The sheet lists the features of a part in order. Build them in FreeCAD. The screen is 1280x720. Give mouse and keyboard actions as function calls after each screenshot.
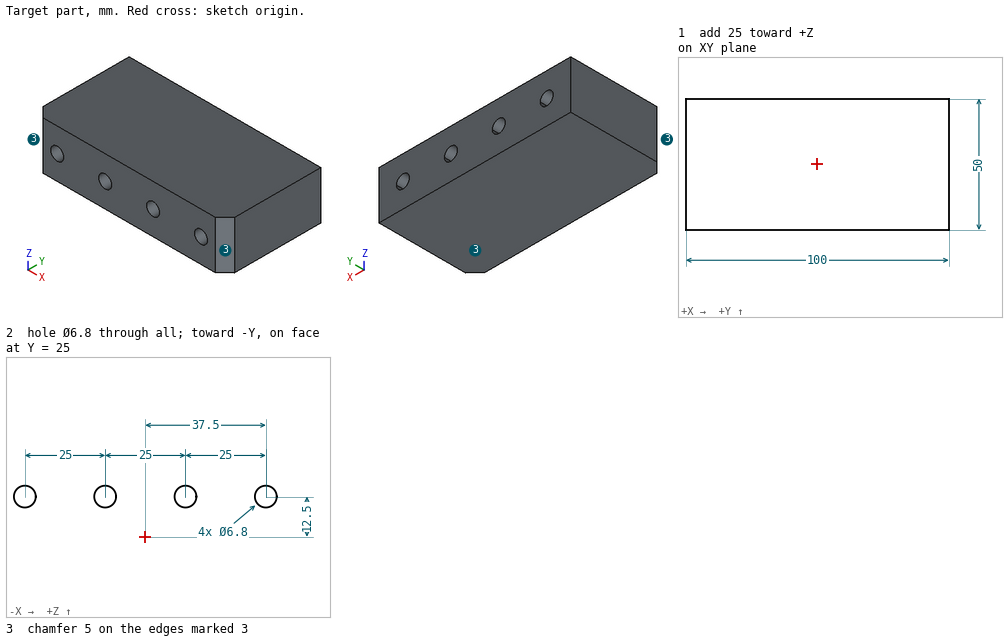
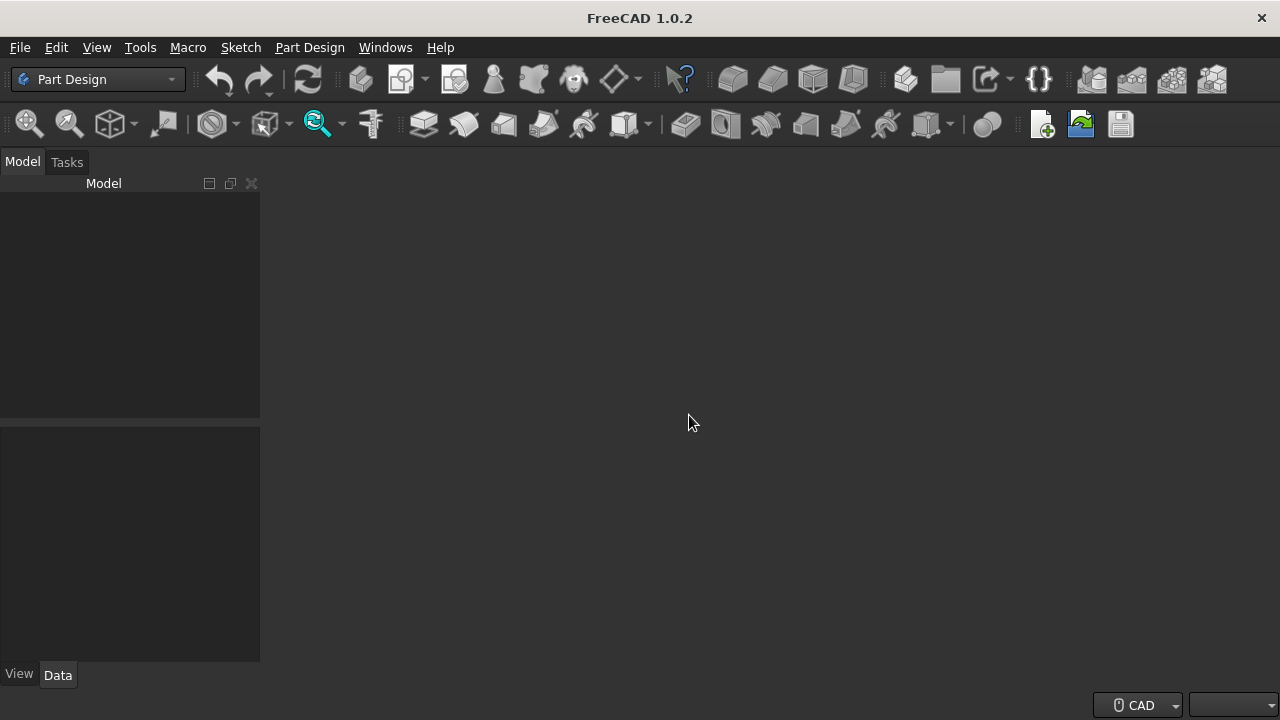
click(1042, 124)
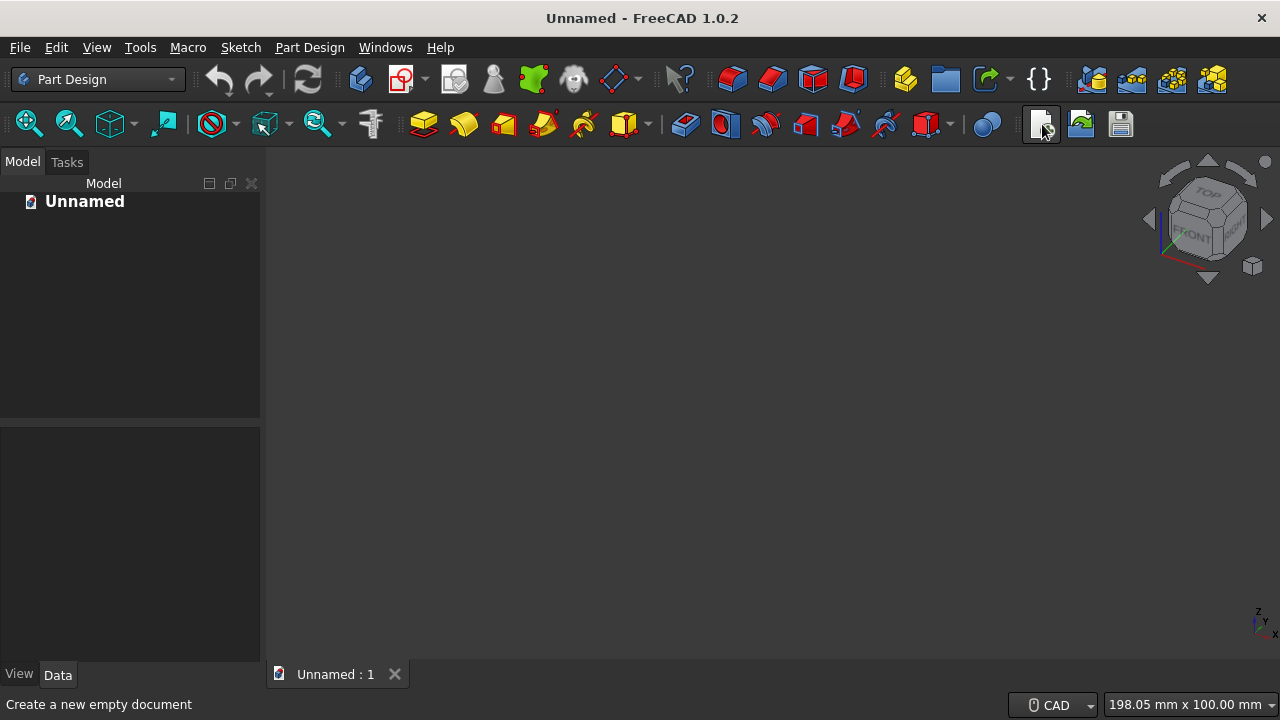
click(402, 80)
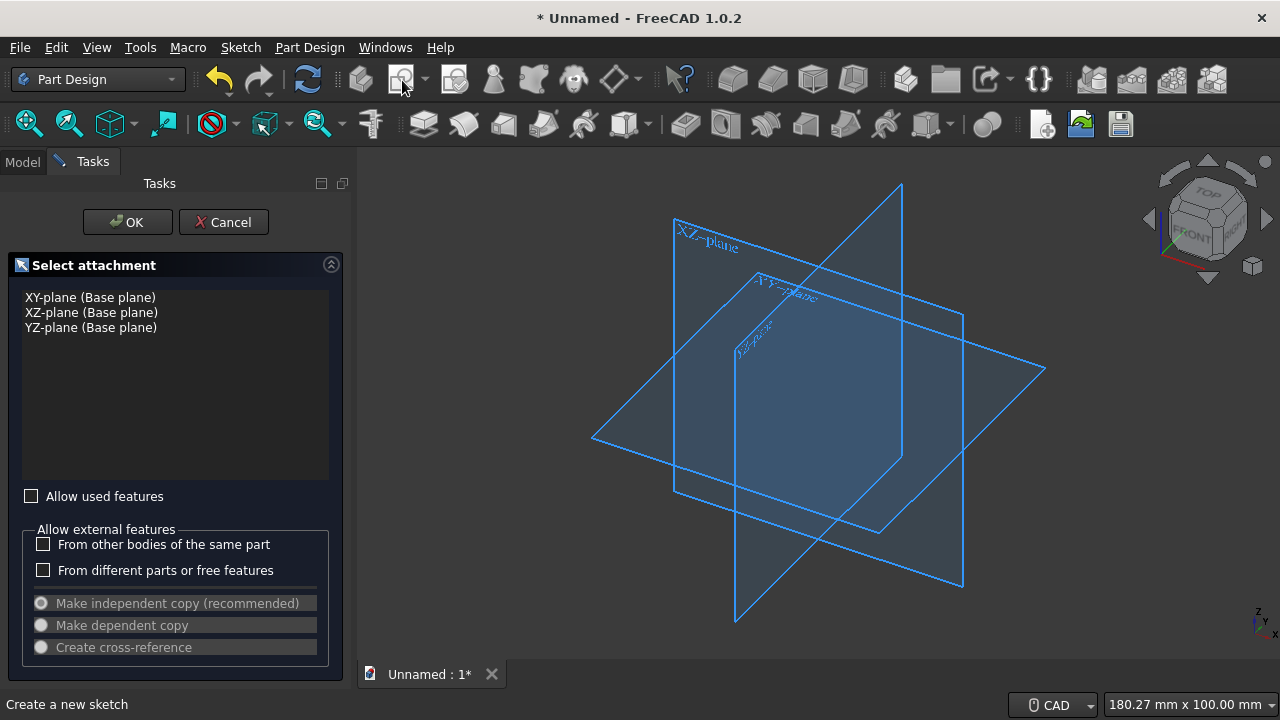
click(82, 298)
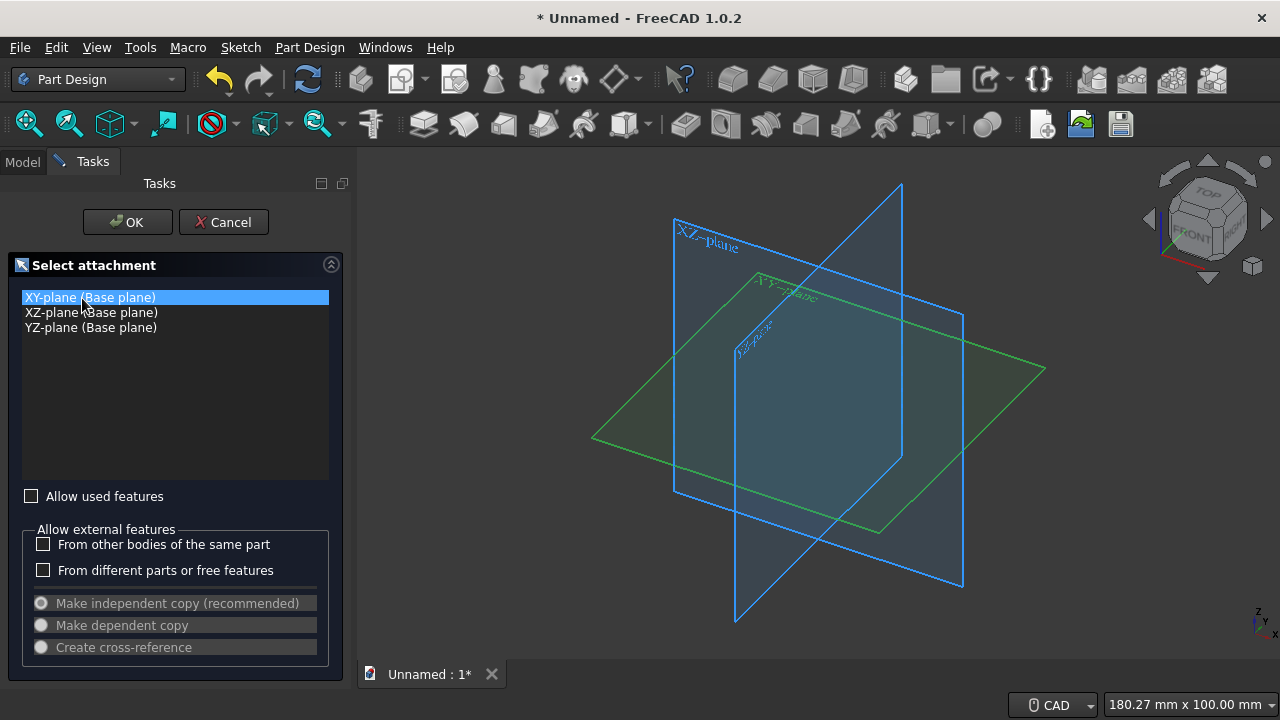
click(128, 222)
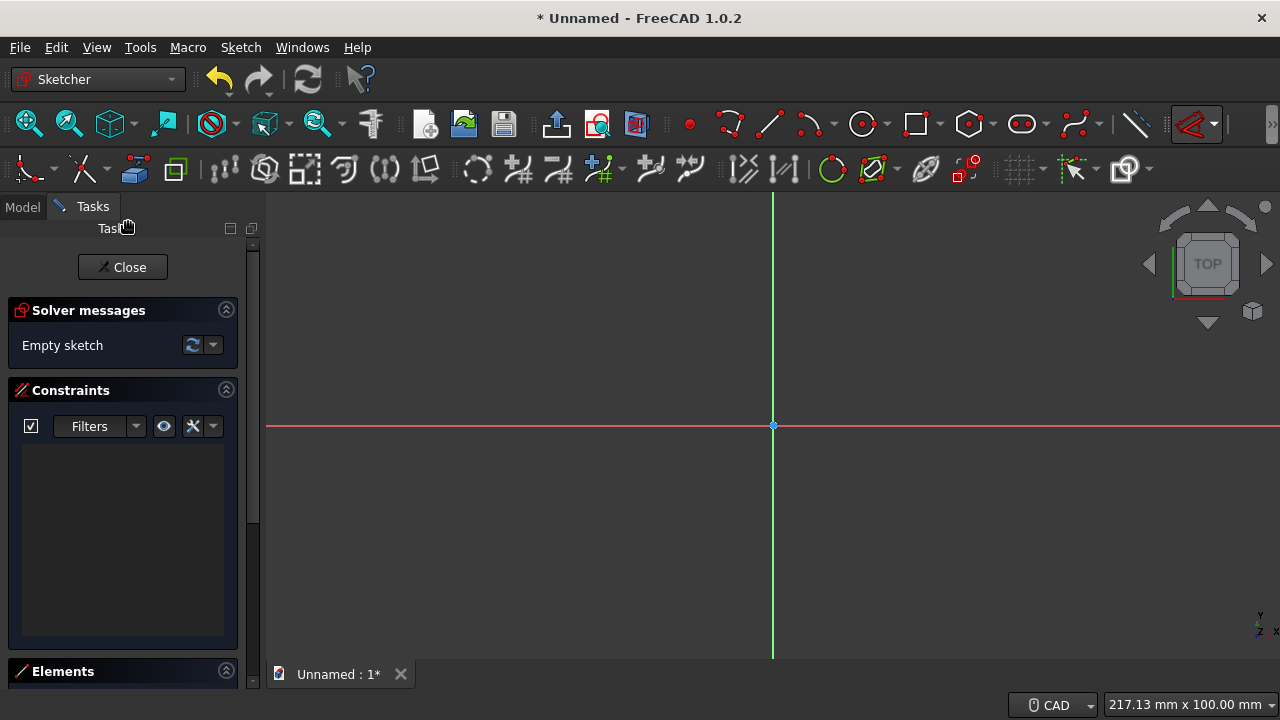
click(942, 124)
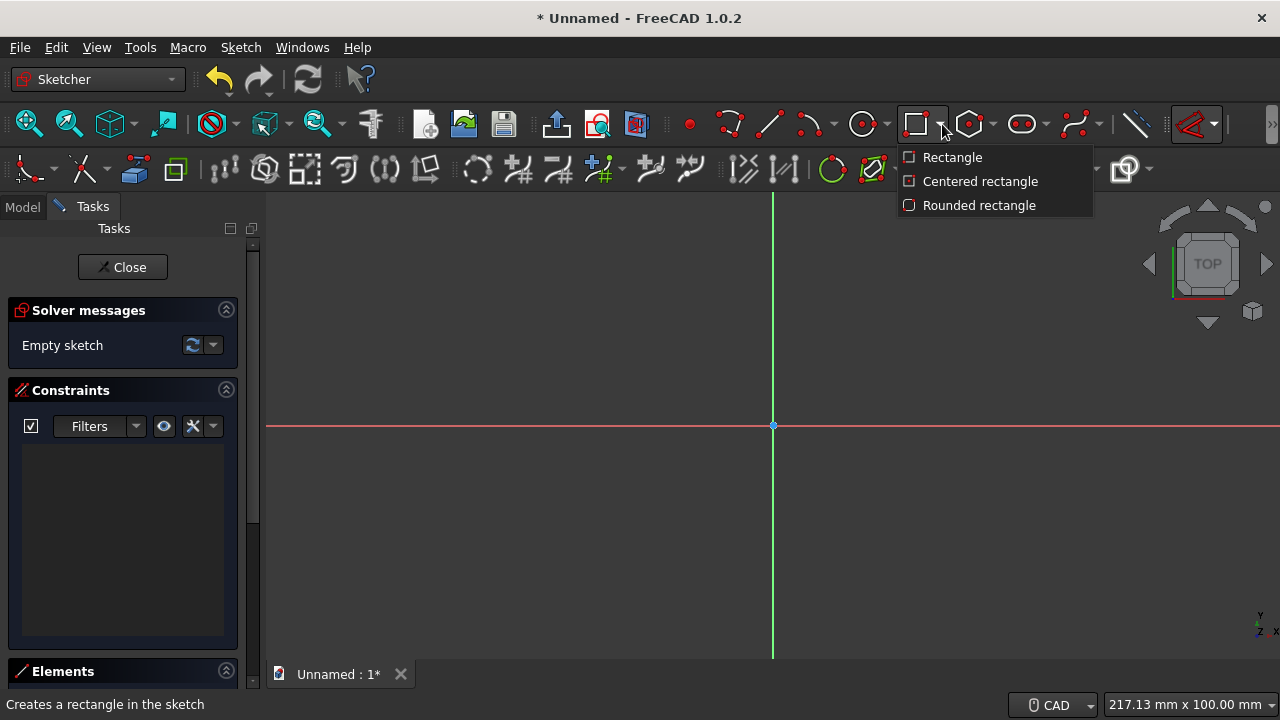
click(996, 181)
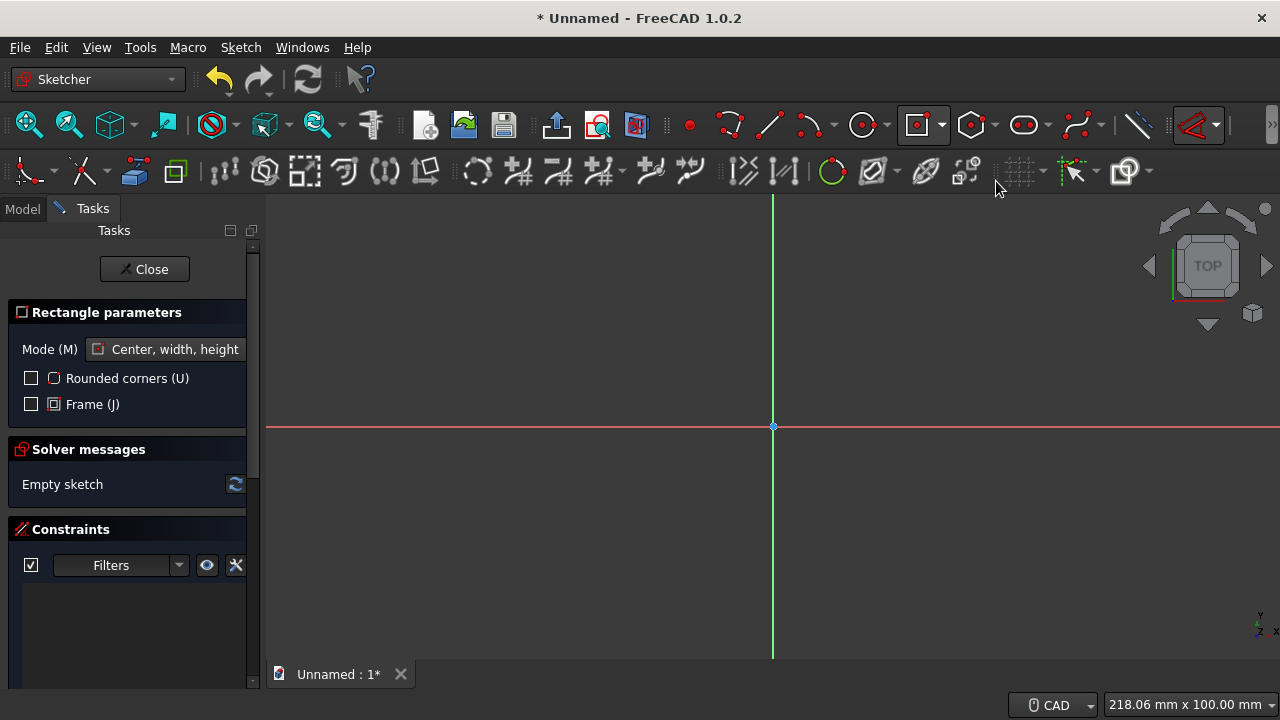
click(773, 426)
move(1006, 310)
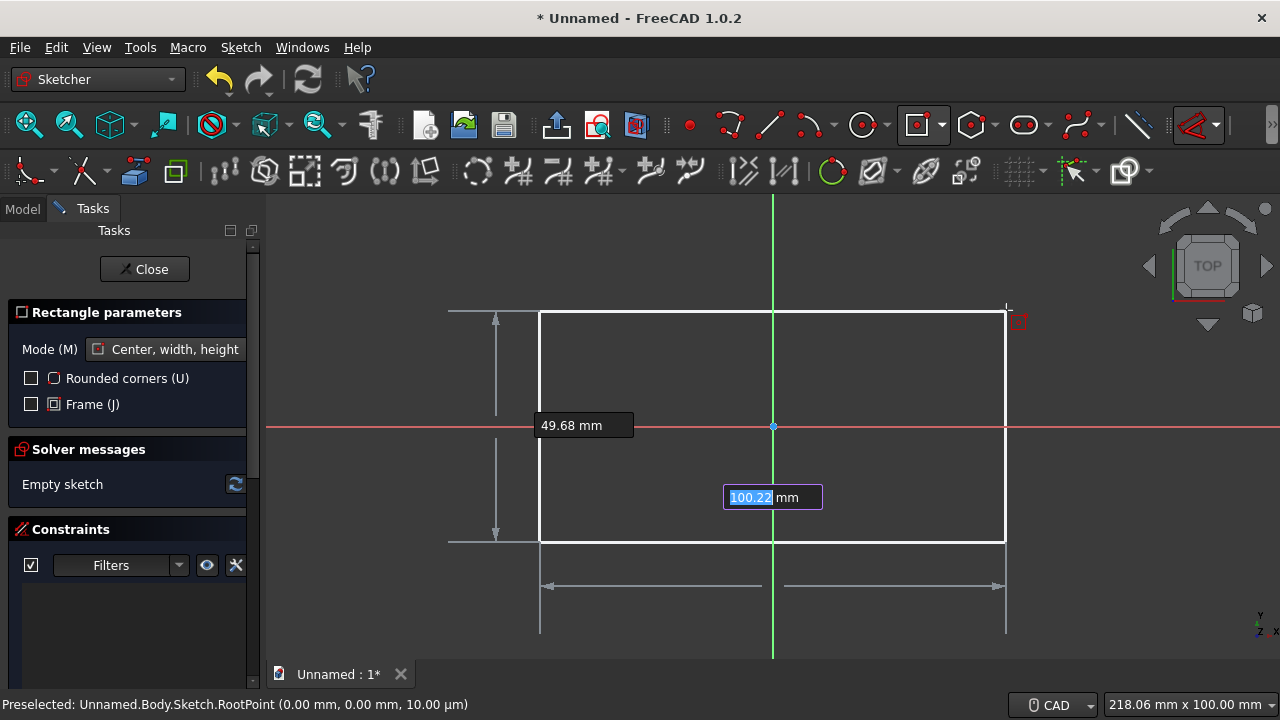
text(100)
key(Tab)
text(50)
key(Return)
key(Escape)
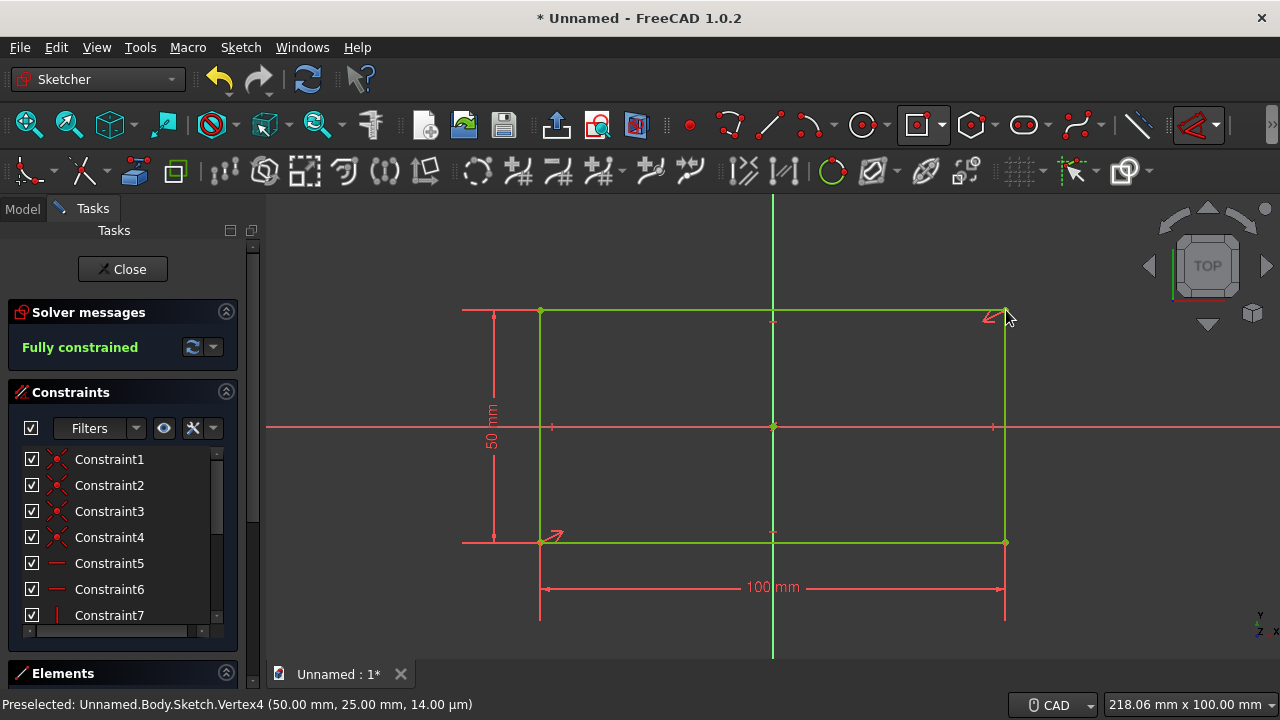
click(123, 269)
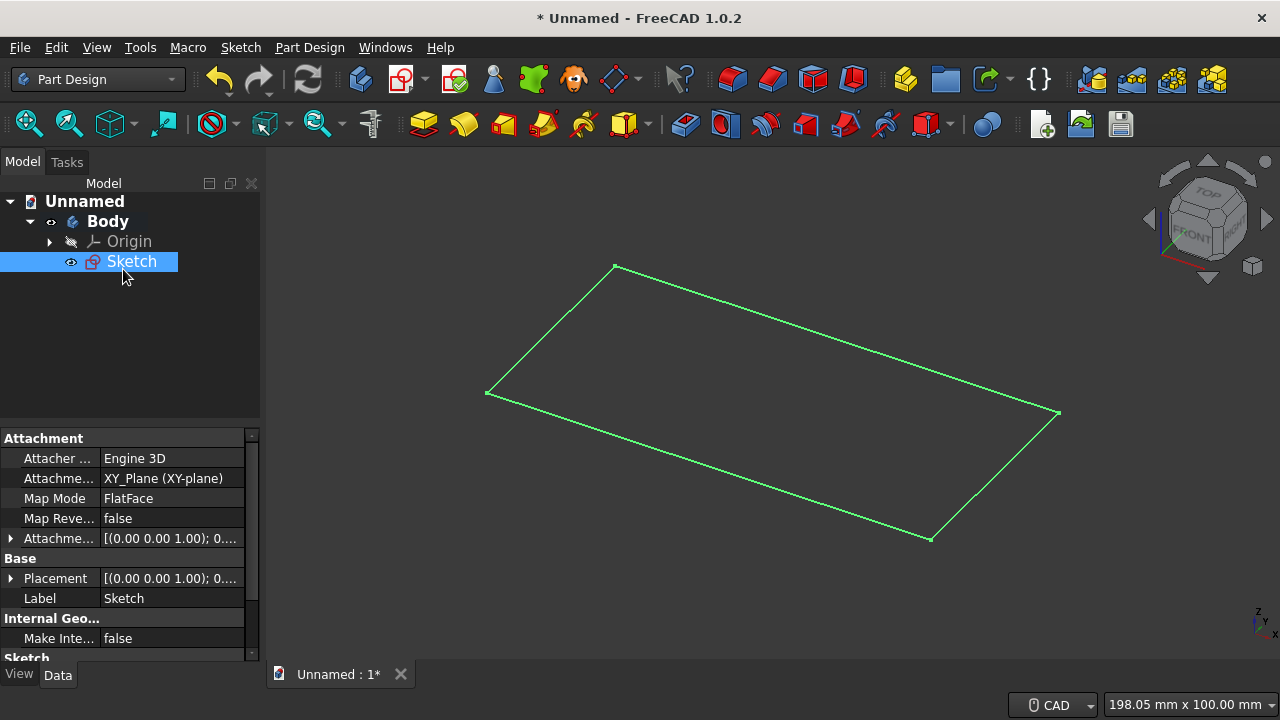
click(424, 124)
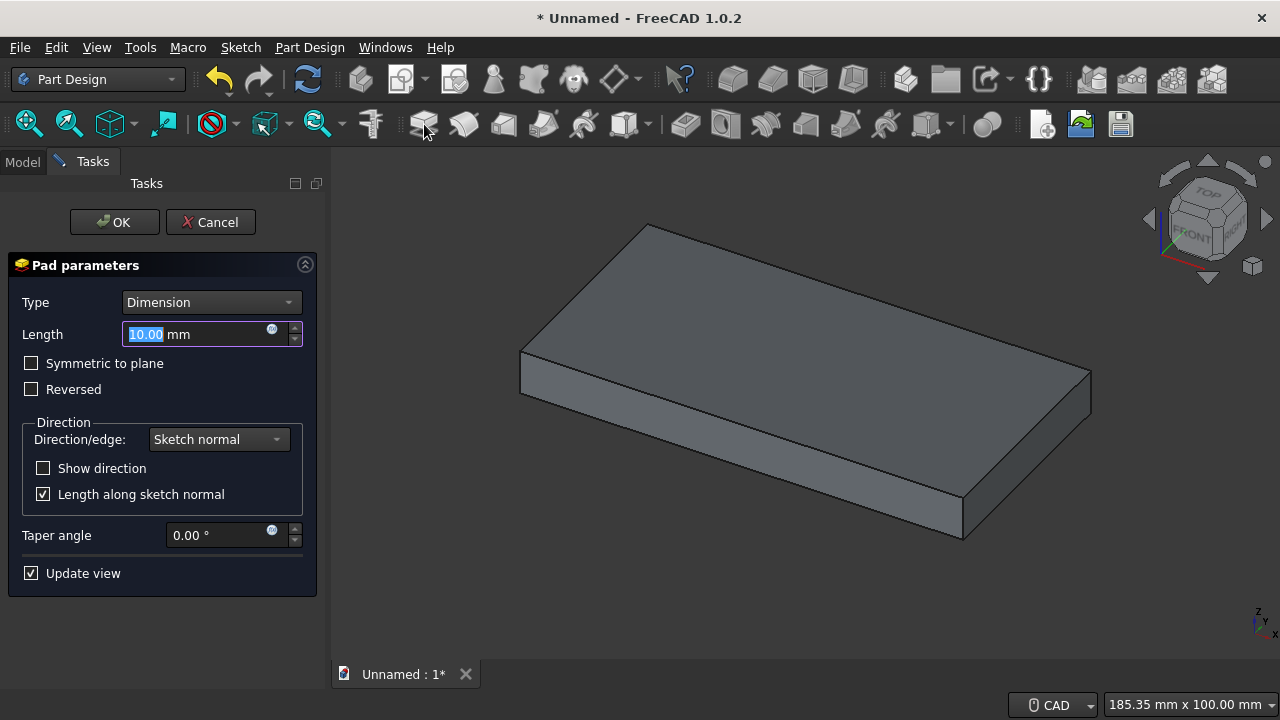
text(25)
key(Tab)